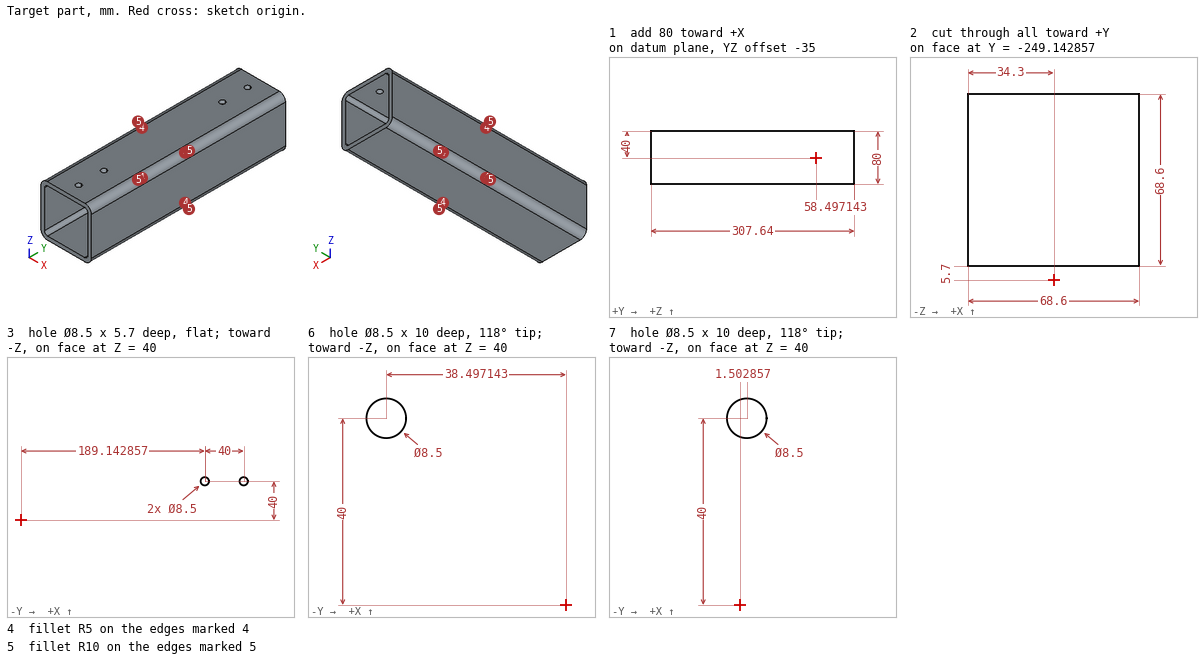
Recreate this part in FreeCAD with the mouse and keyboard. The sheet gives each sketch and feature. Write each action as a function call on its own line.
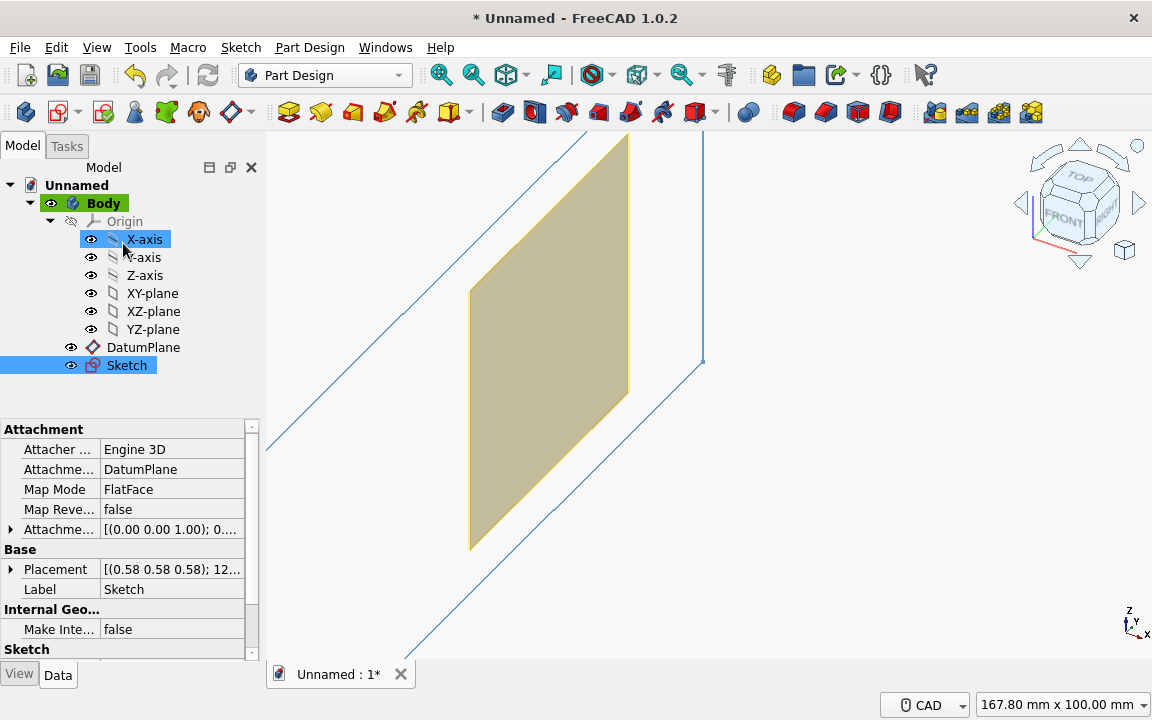
click(290, 112)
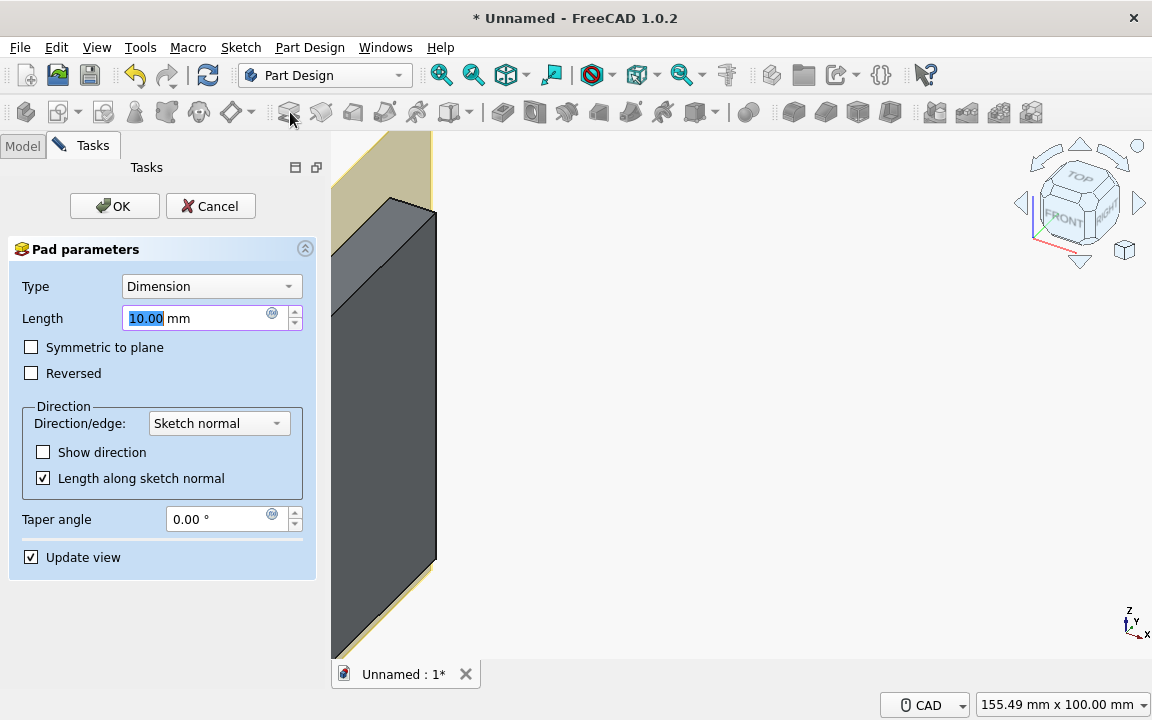
text(80)
key(Tab)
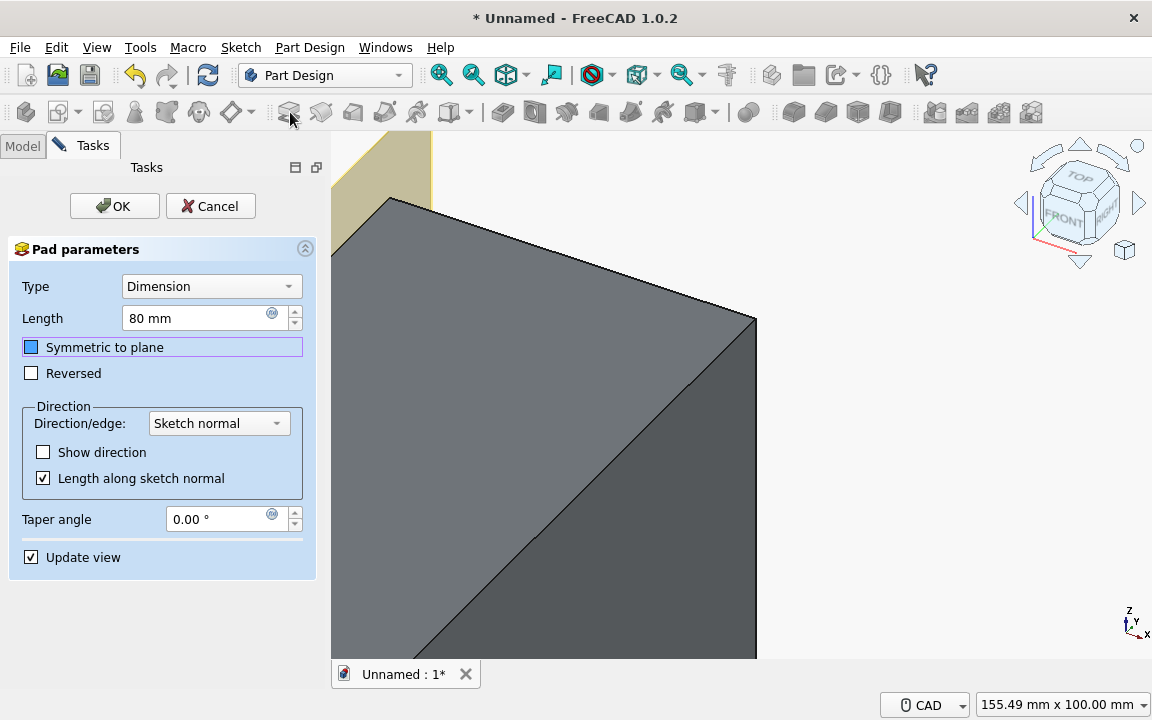
click(115, 206)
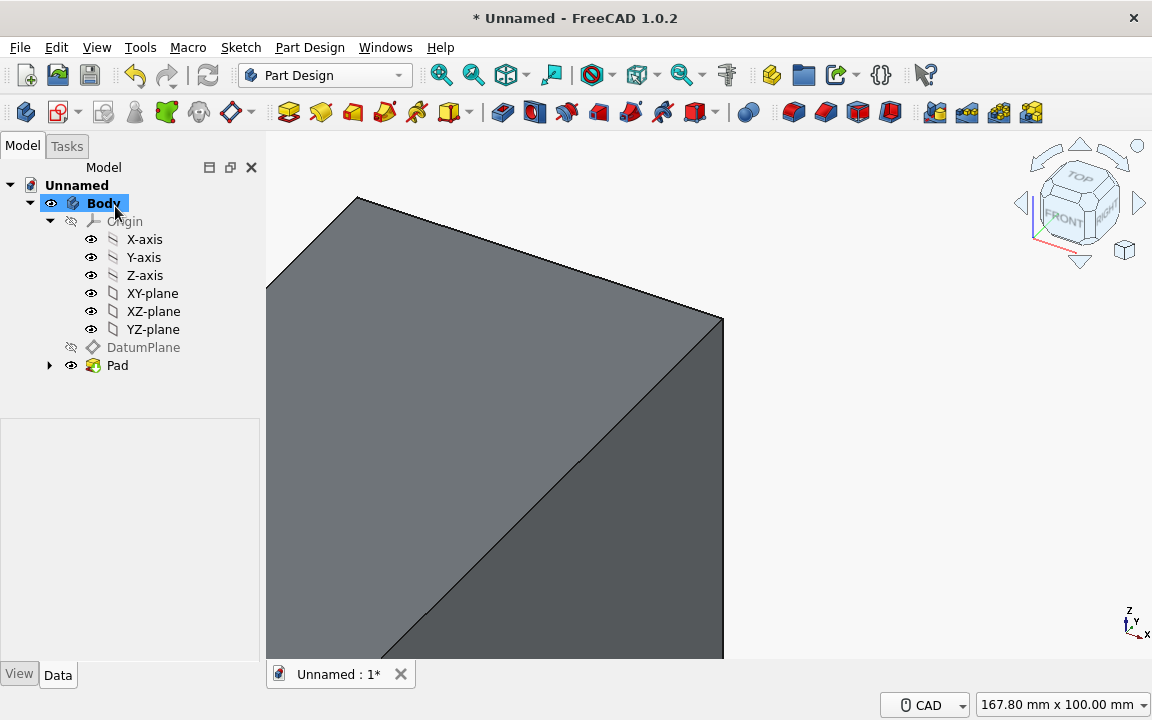
click(442, 76)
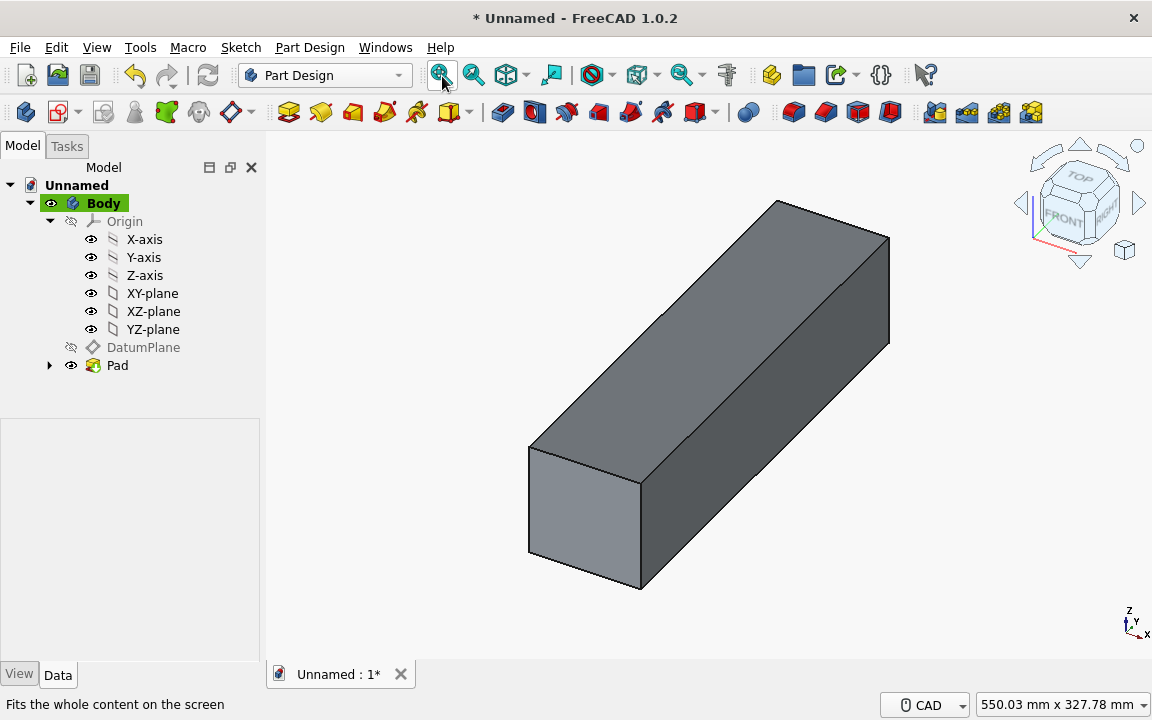
click(585, 517)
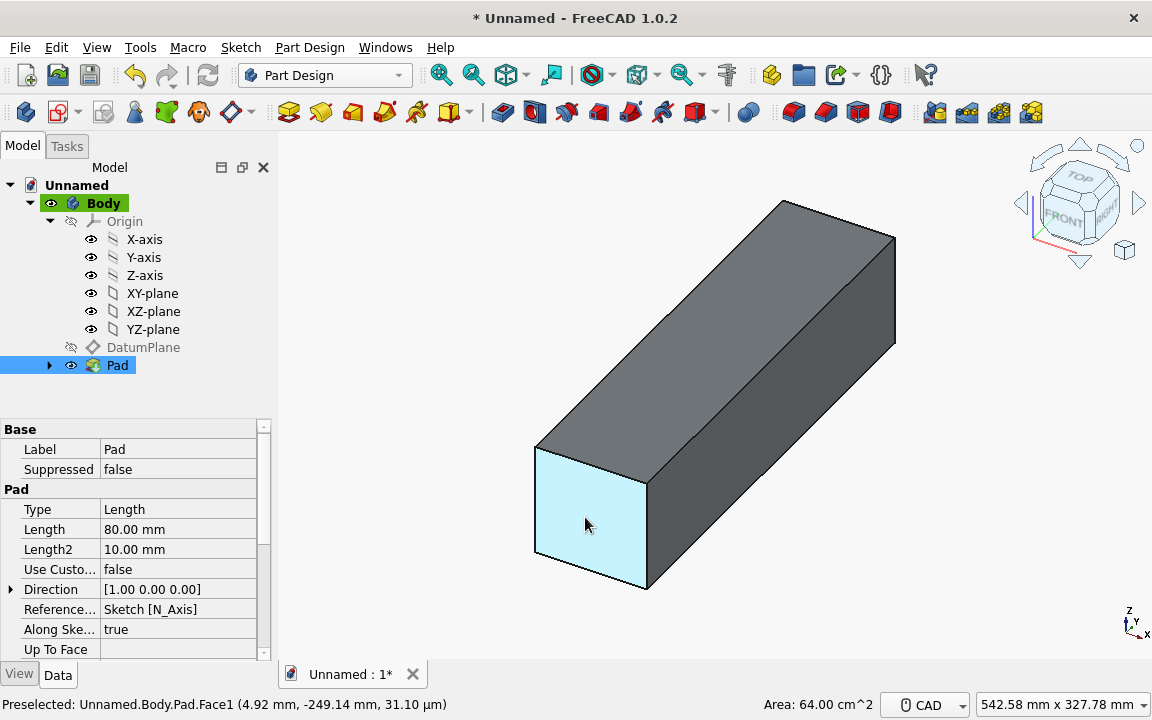
click(58, 112)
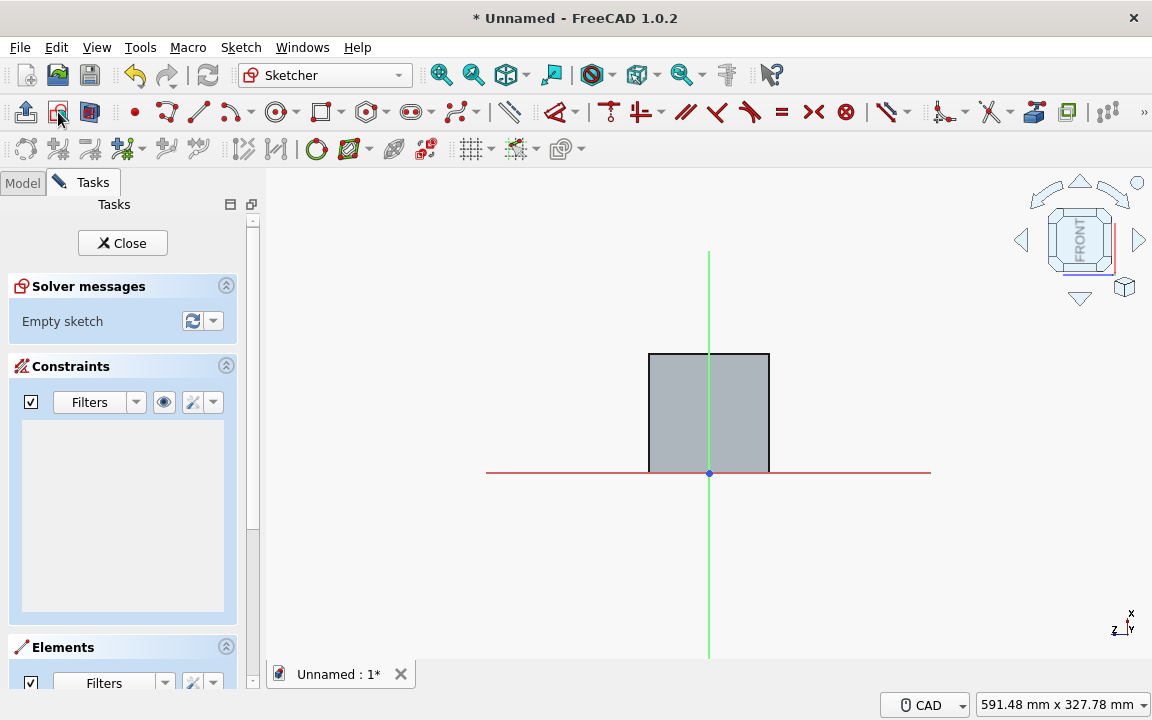
scroll(749, 420, up, 5)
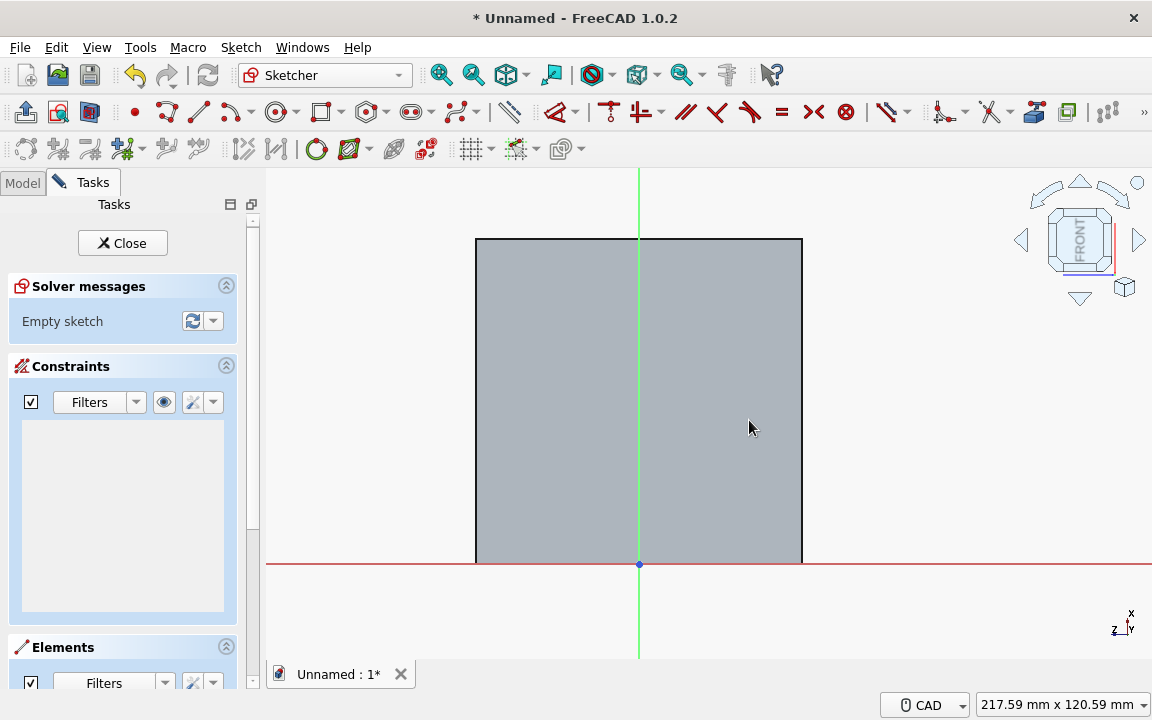
click(322, 112)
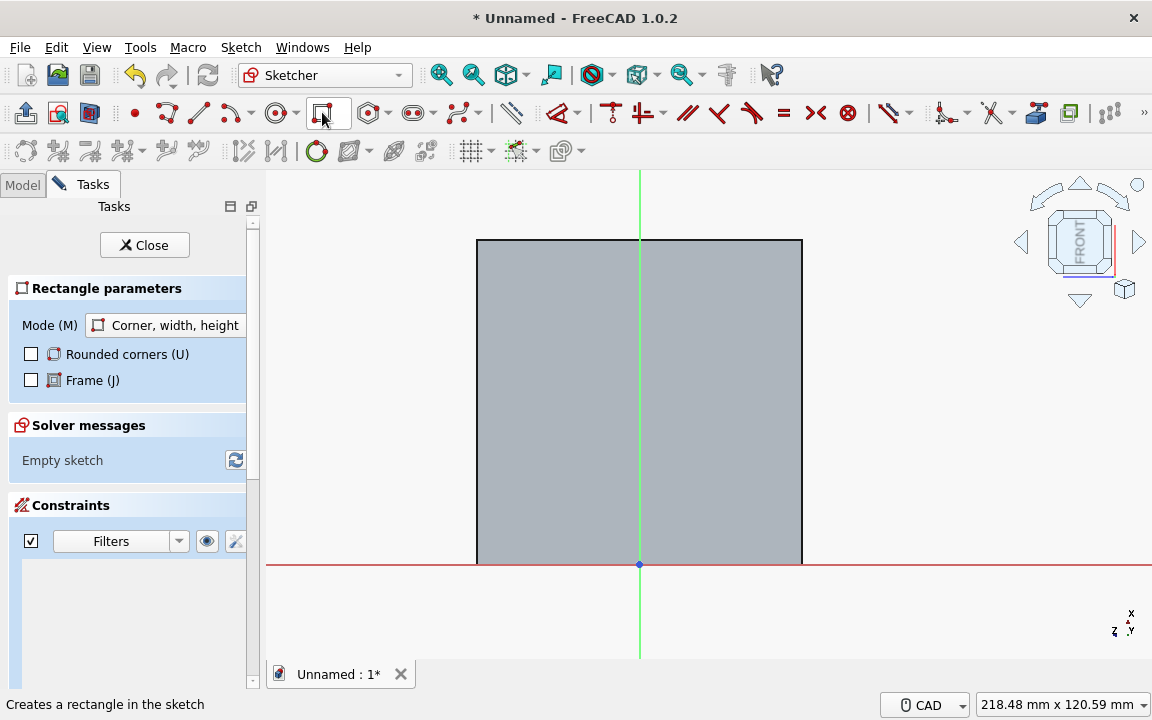
click(501, 263)
move(779, 542)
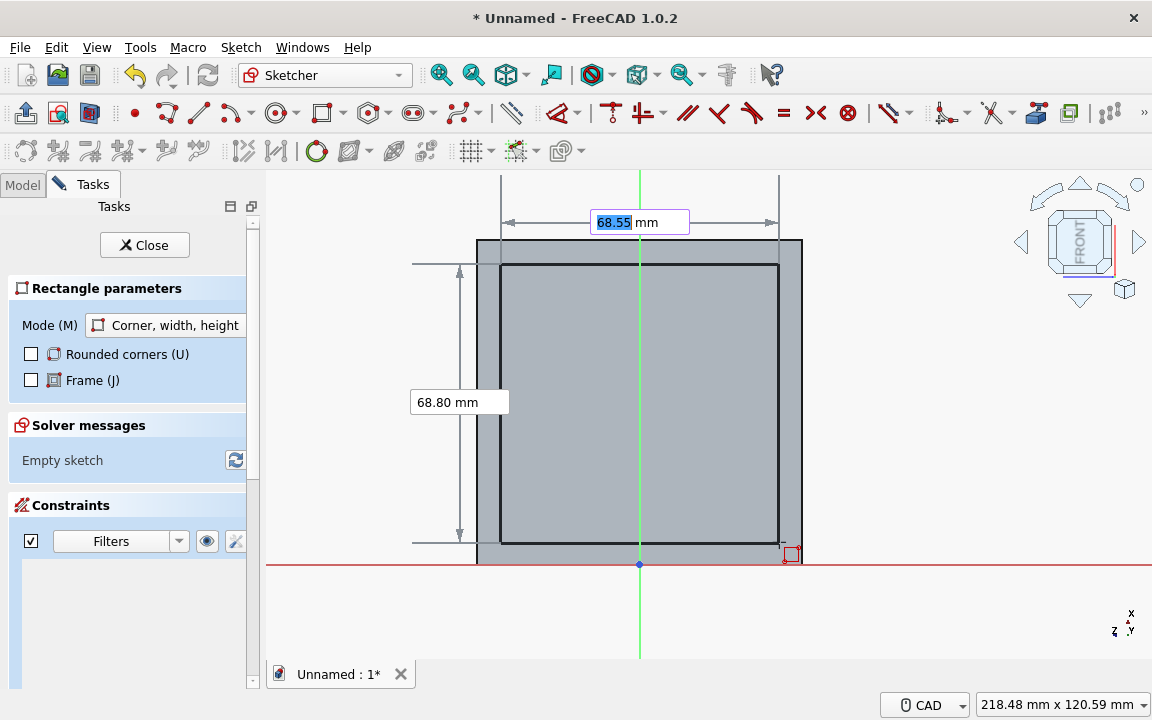
text(68.6)
key(Tab)
text(68.6)
key(Return)
key(Escape)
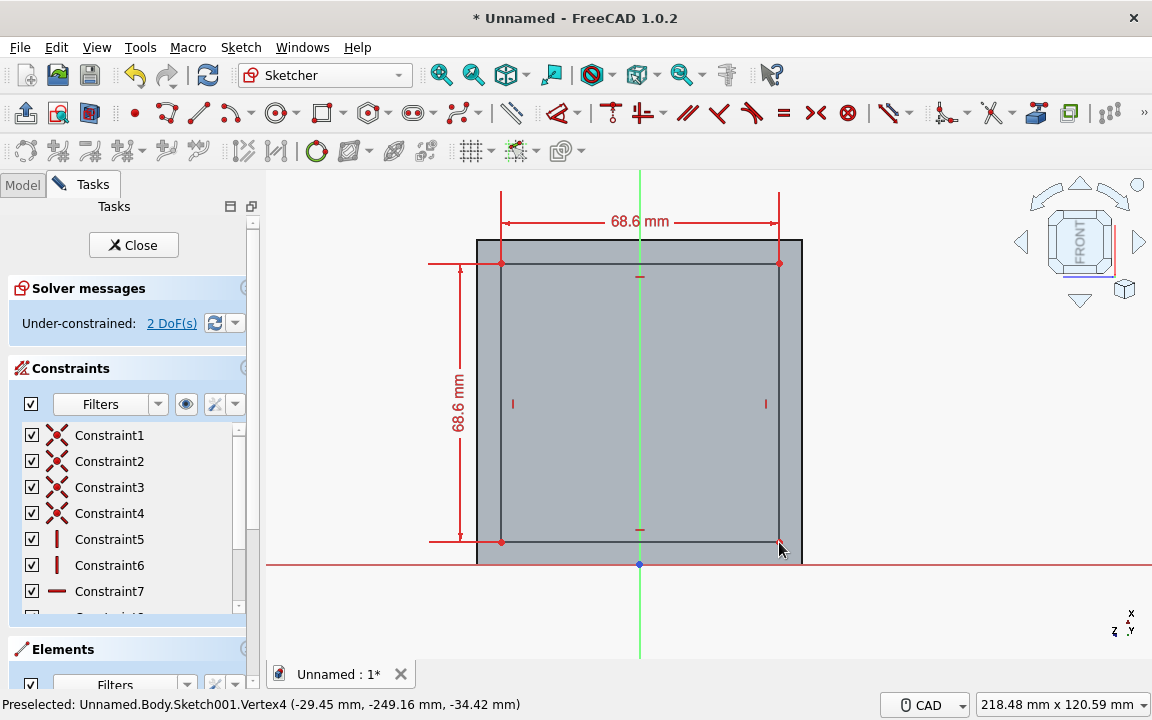
scroll(501, 542, up, 3)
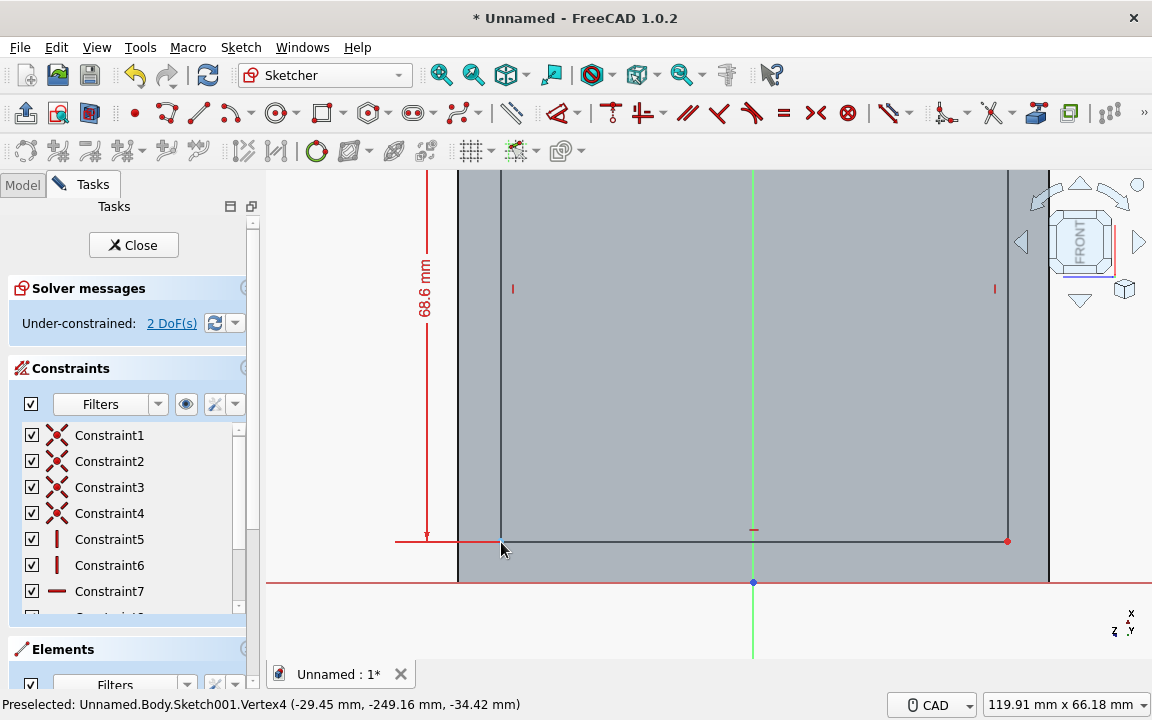
click(501, 542)